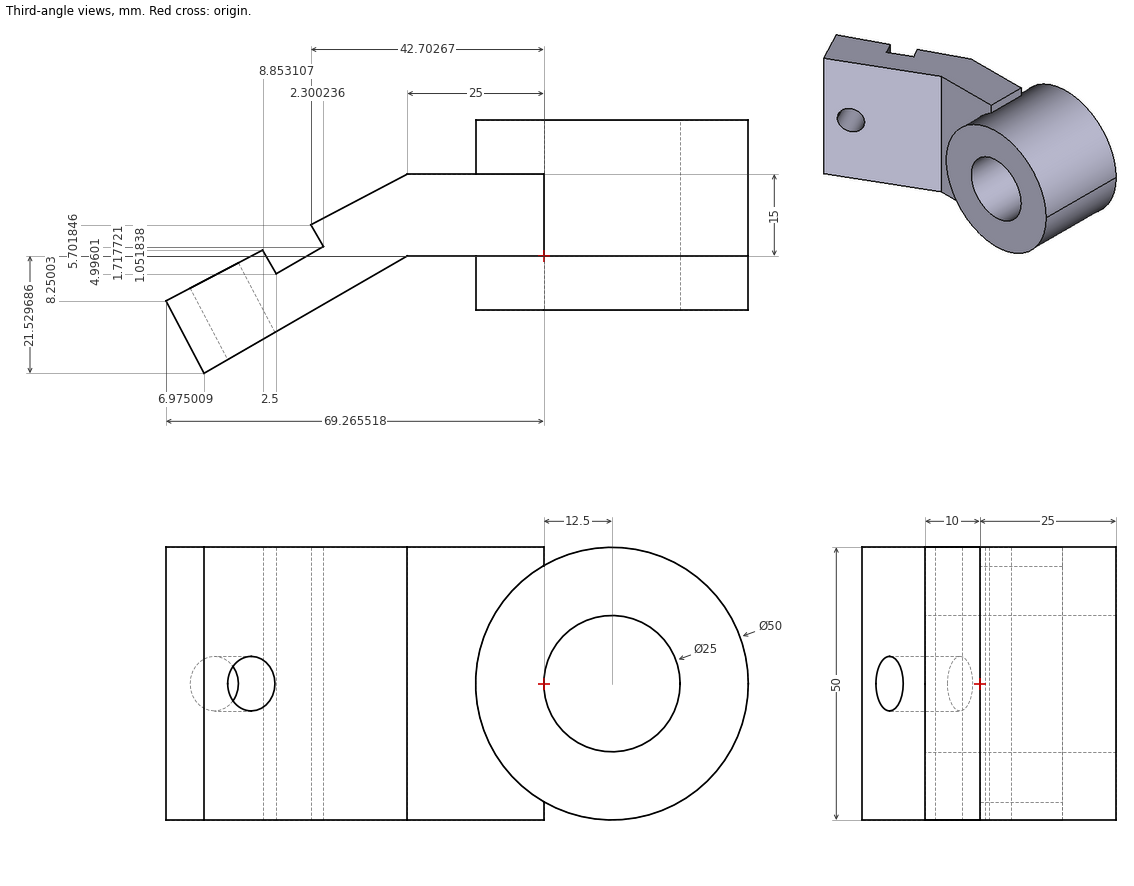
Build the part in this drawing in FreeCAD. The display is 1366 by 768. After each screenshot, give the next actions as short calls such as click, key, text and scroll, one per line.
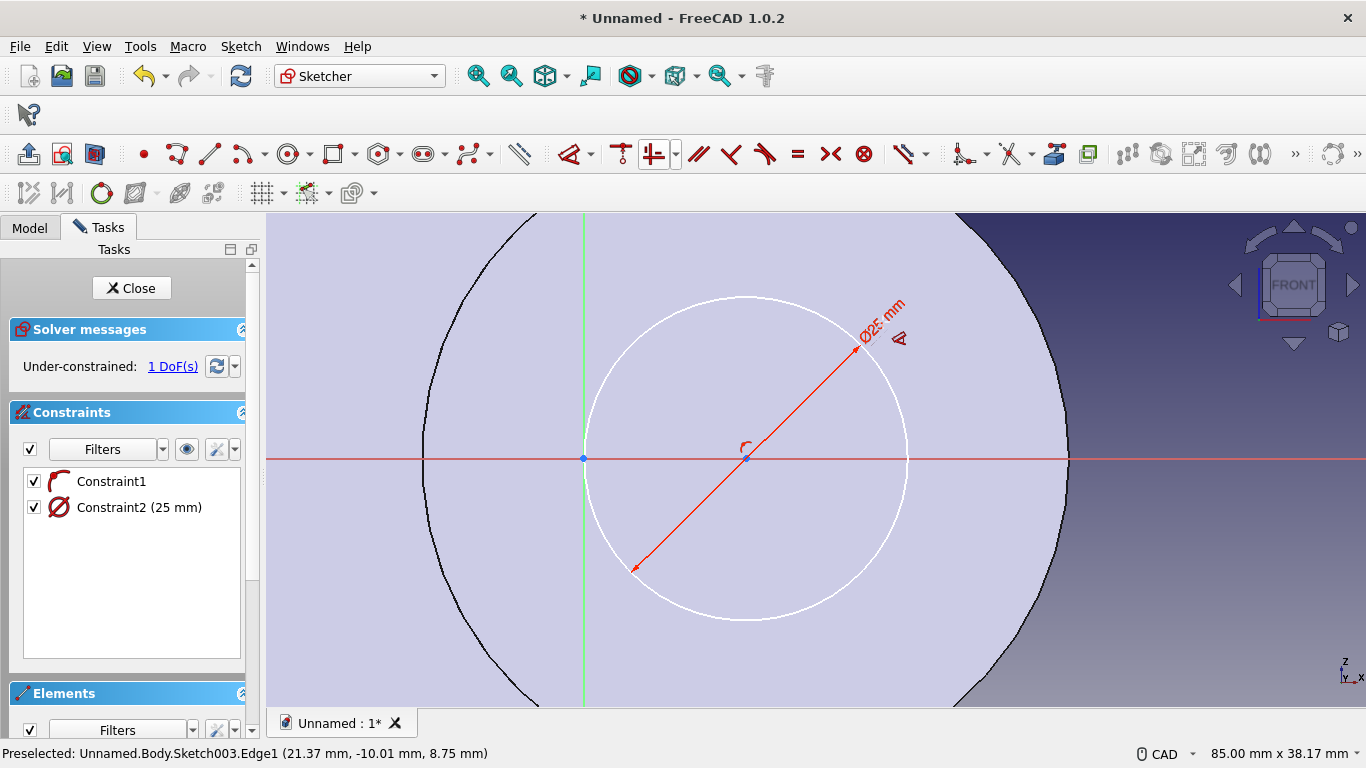
click(746, 459)
click(665, 493)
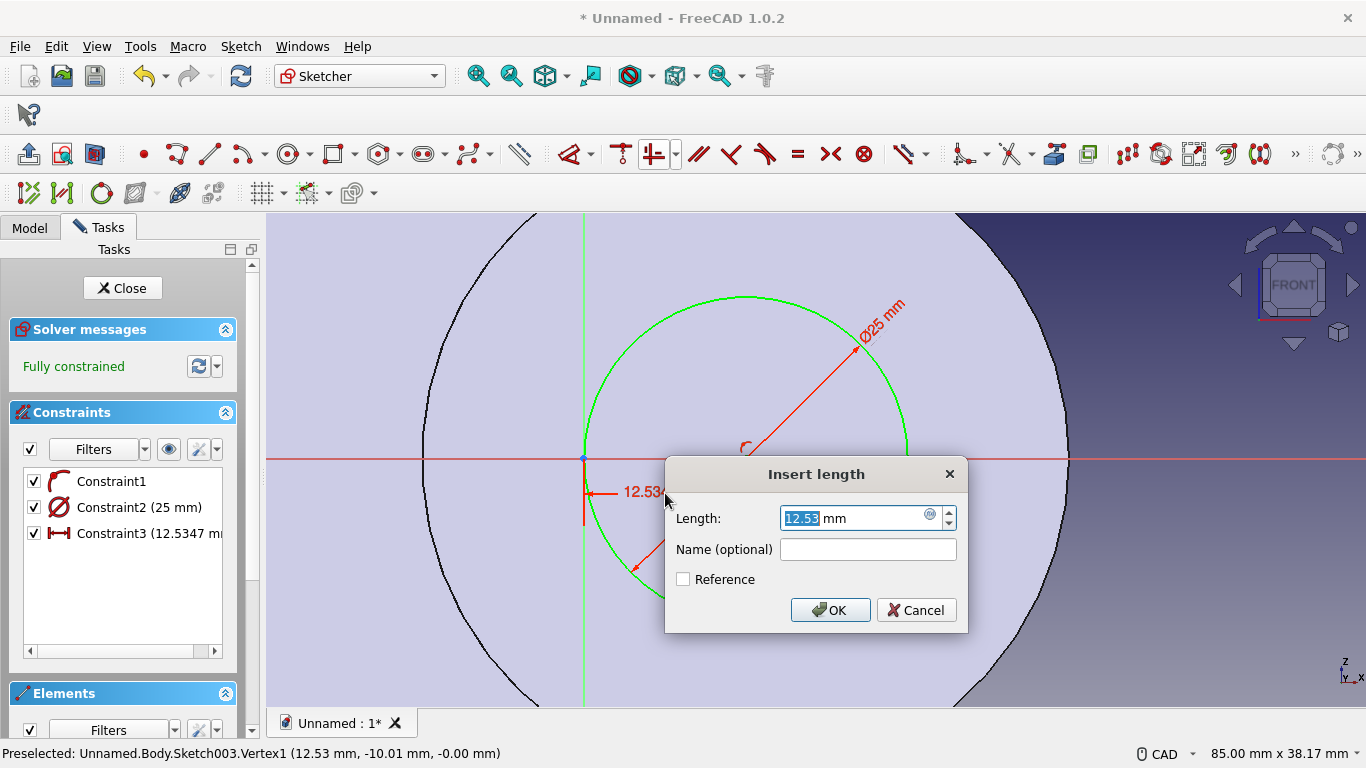
text(12.5)
key(Return)
key(Escape)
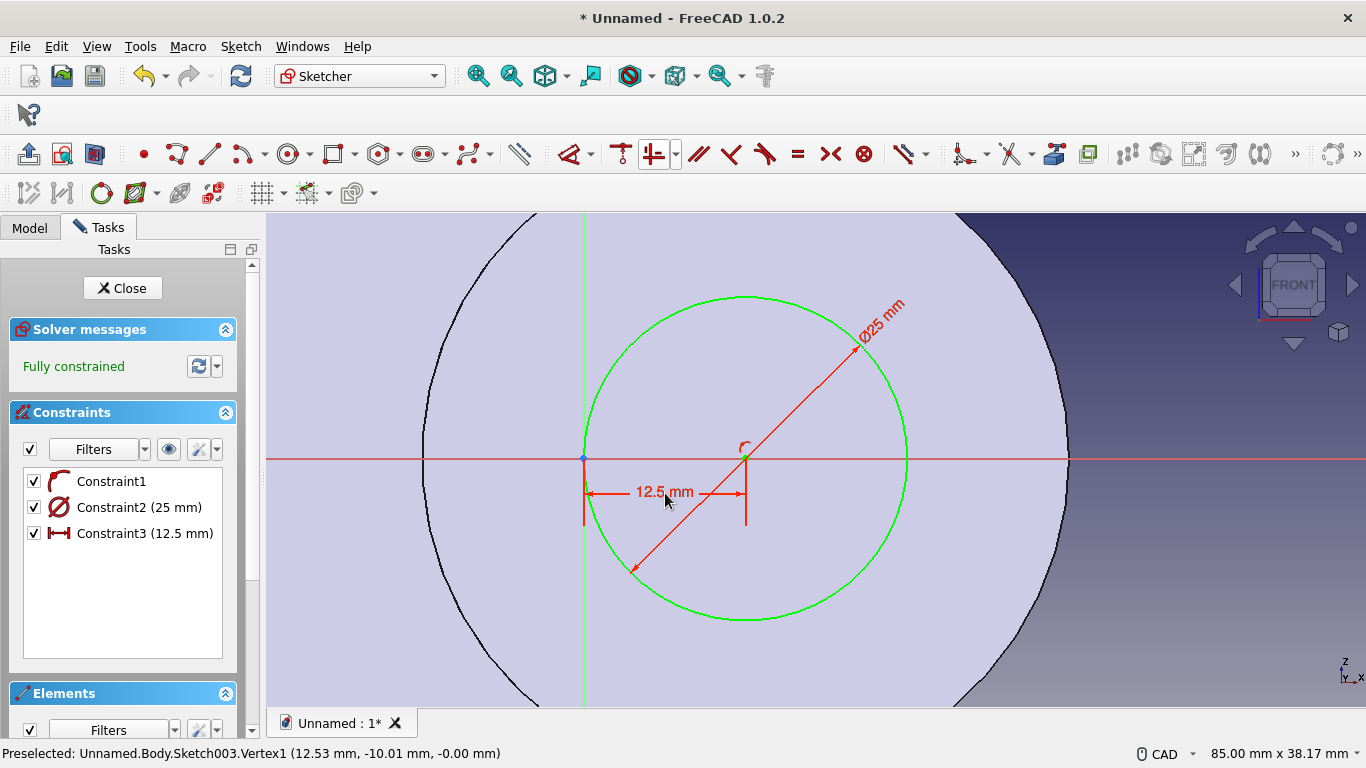
click(123, 288)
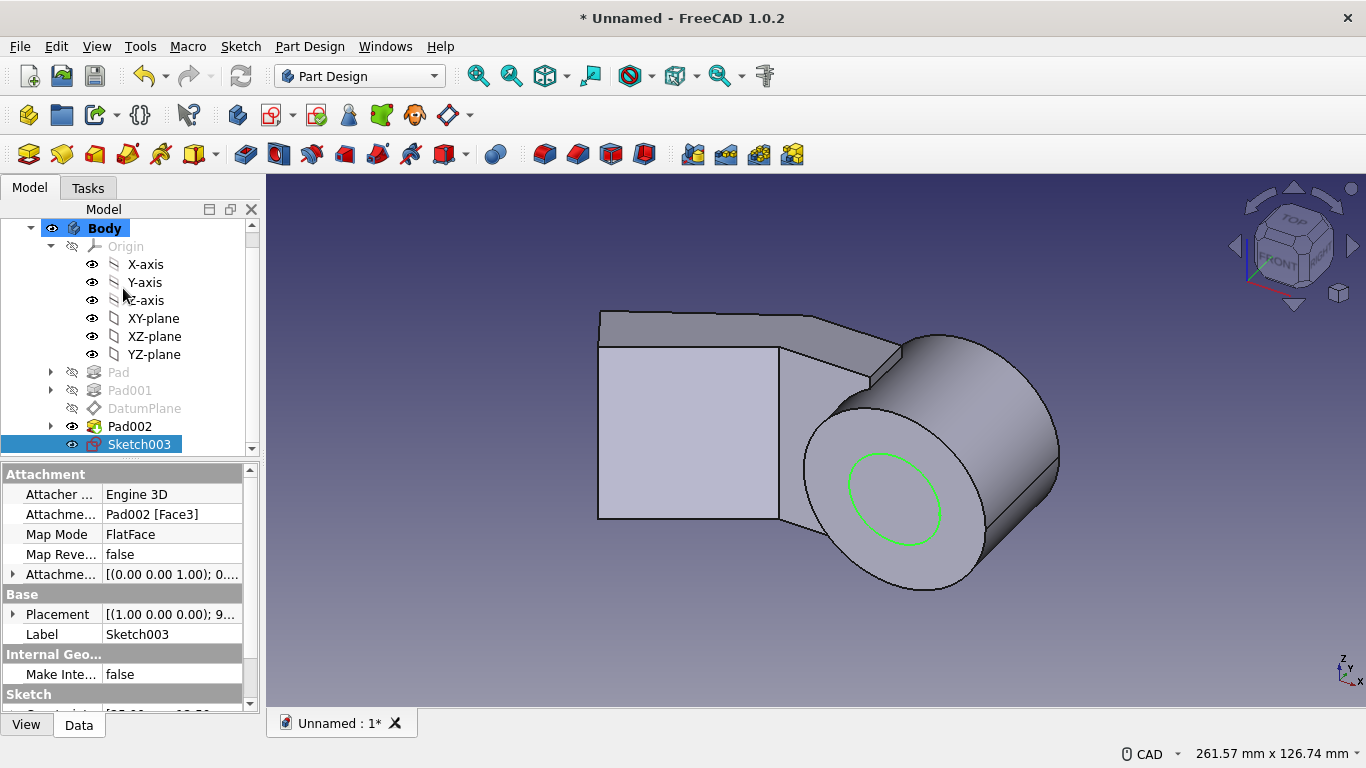
click(246, 154)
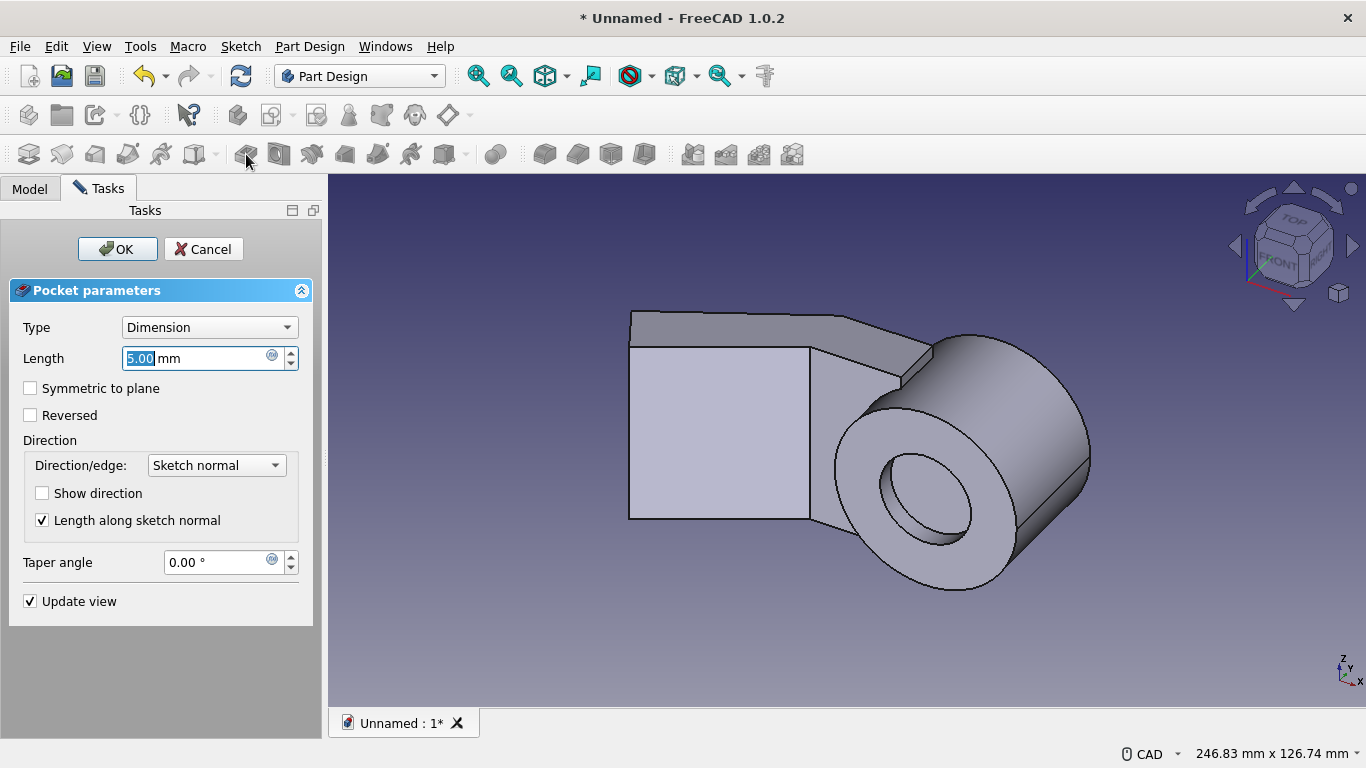
click(210, 328)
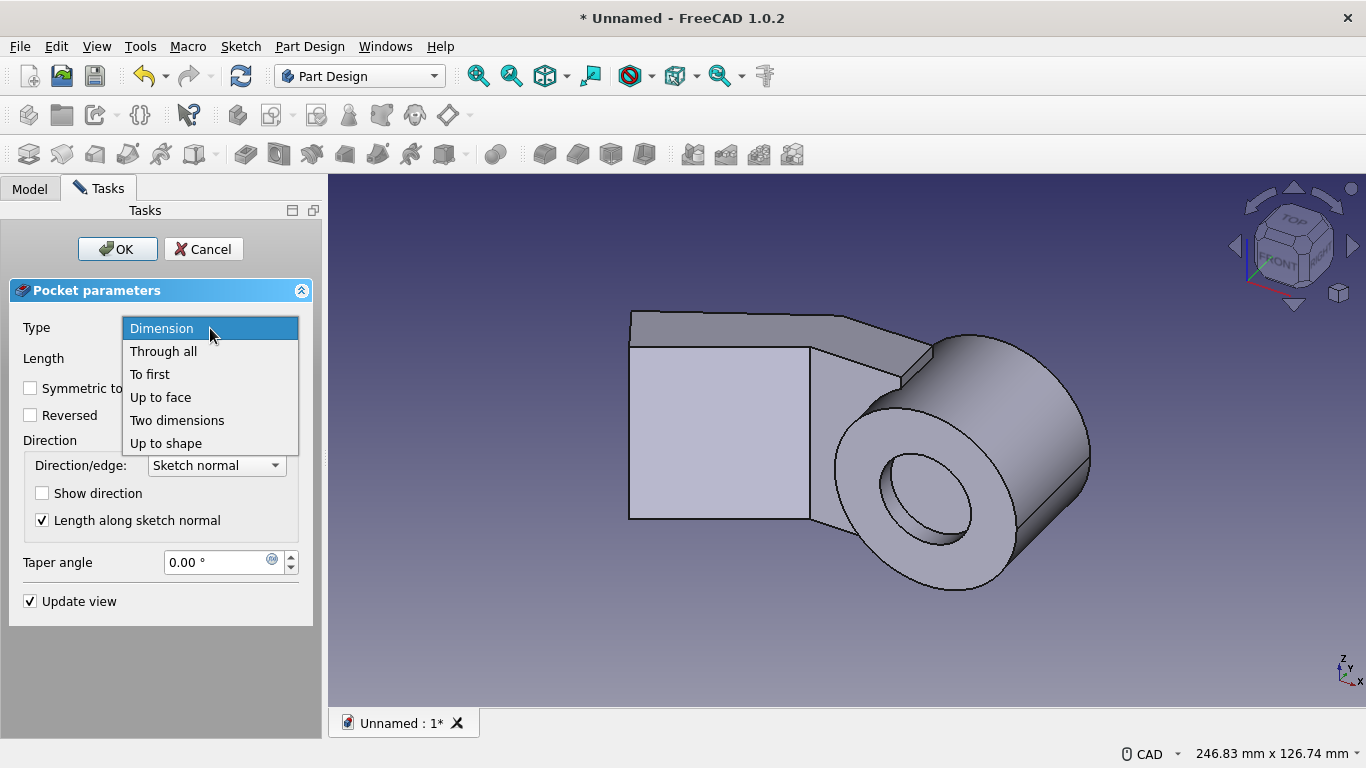
click(208, 352)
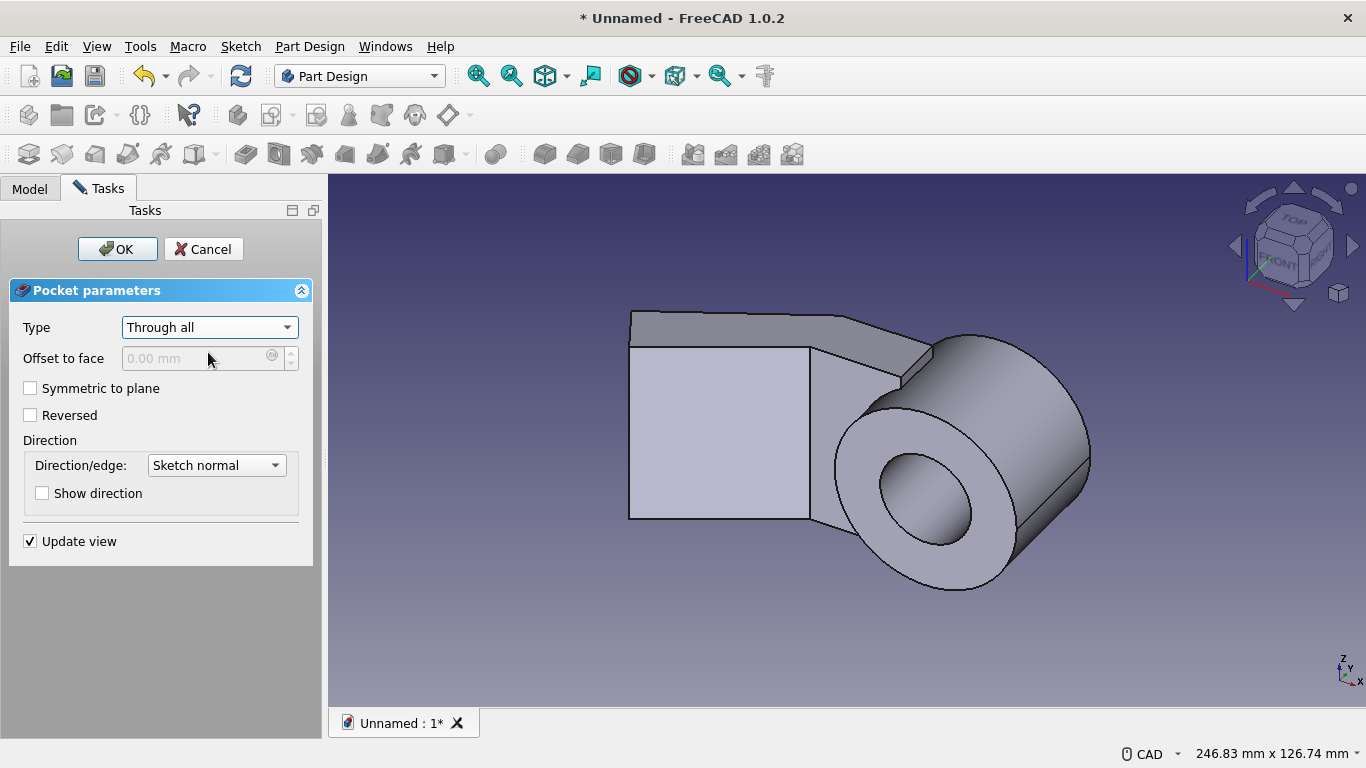
click(118, 249)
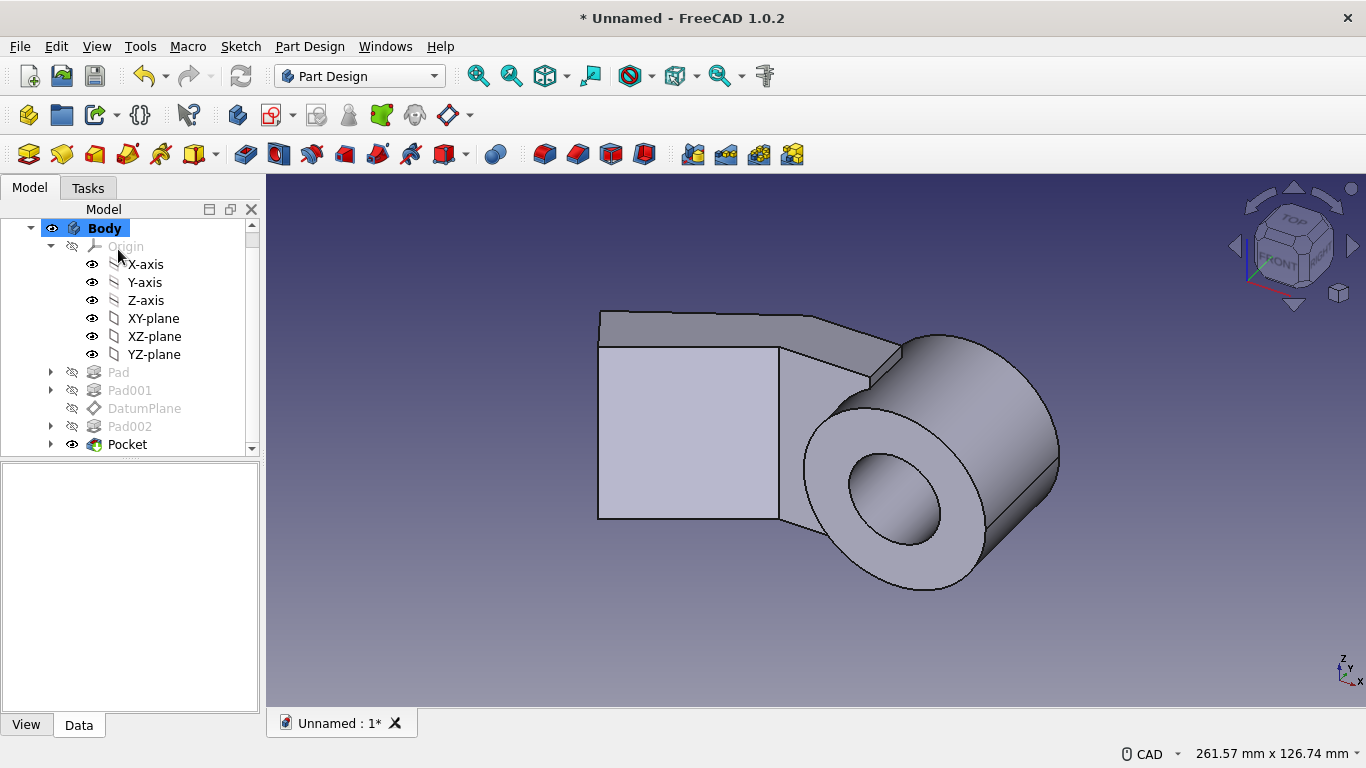
click(831, 343)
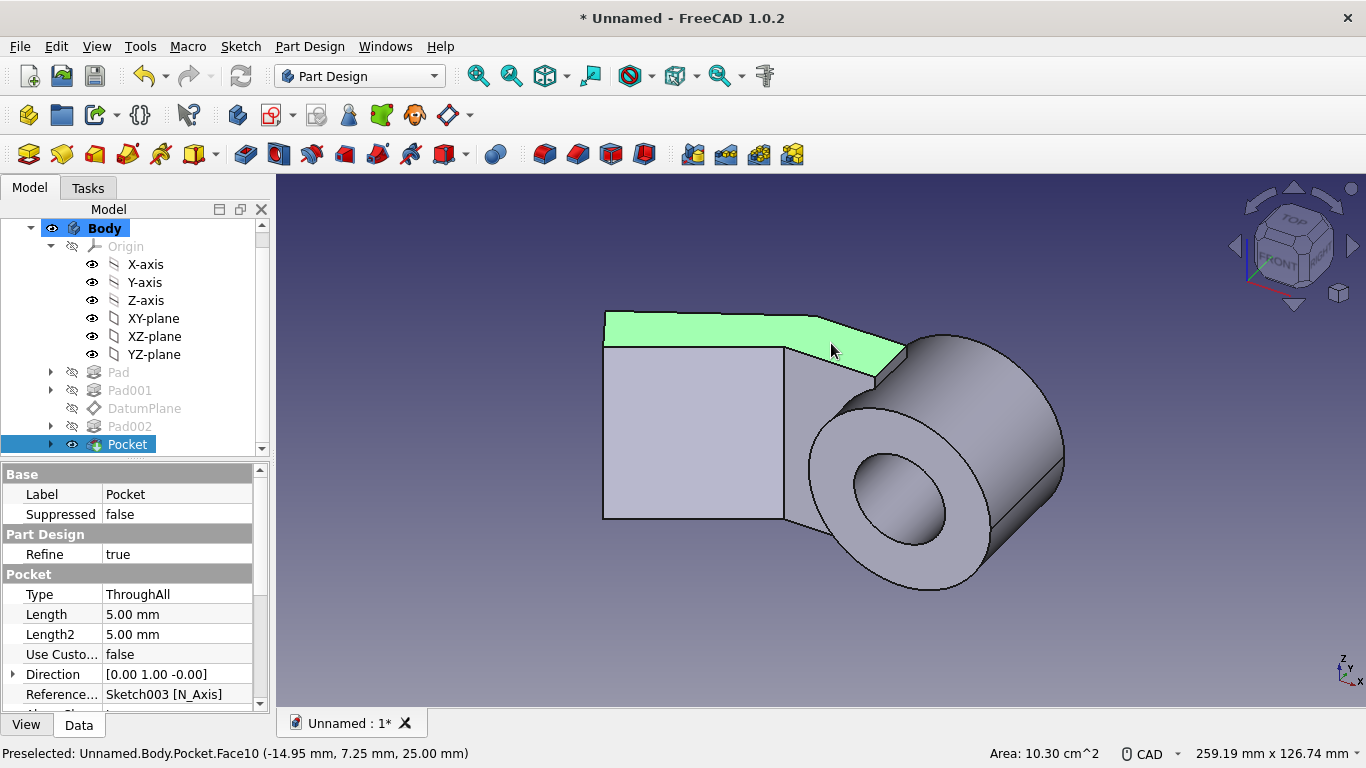
click(270, 116)